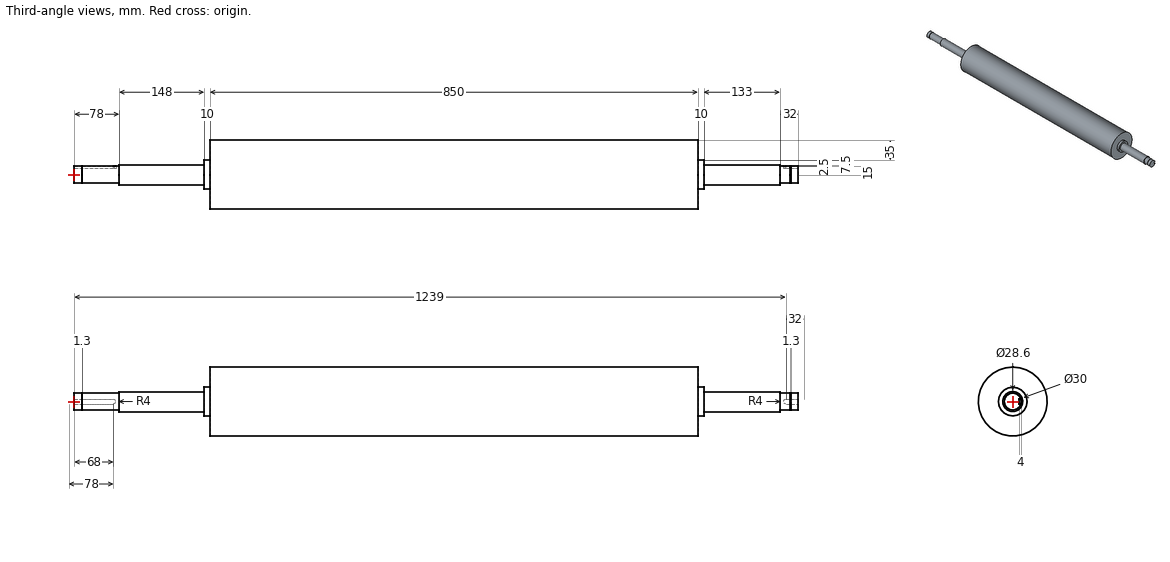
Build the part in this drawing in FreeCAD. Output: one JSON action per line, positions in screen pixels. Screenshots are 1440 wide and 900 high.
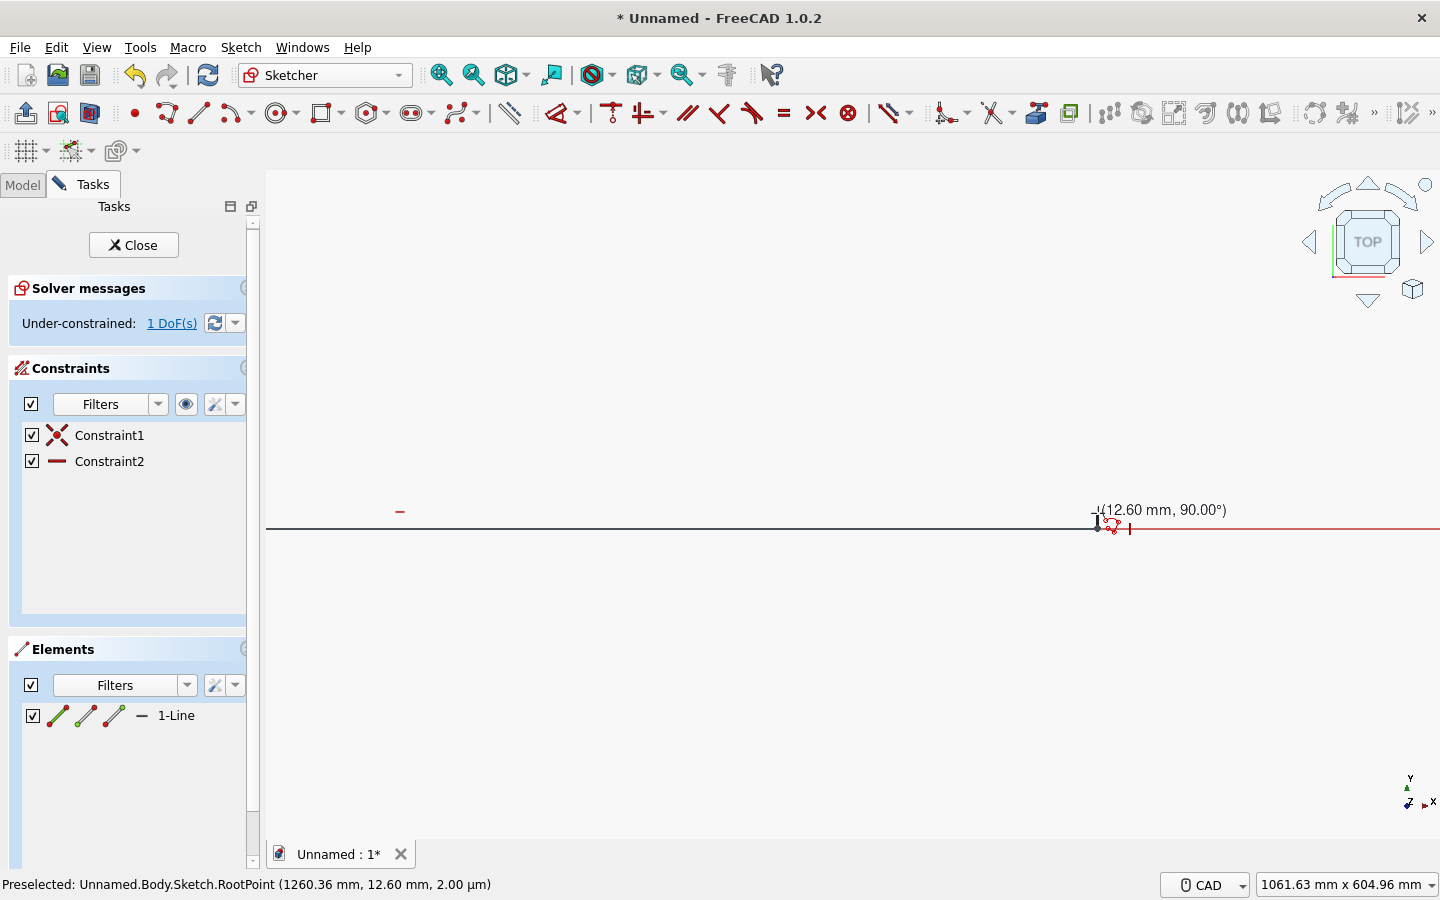
{"action": "left_click", "coordinate": [1097, 512]}
{"action": "left_click", "coordinate": [1062, 512]}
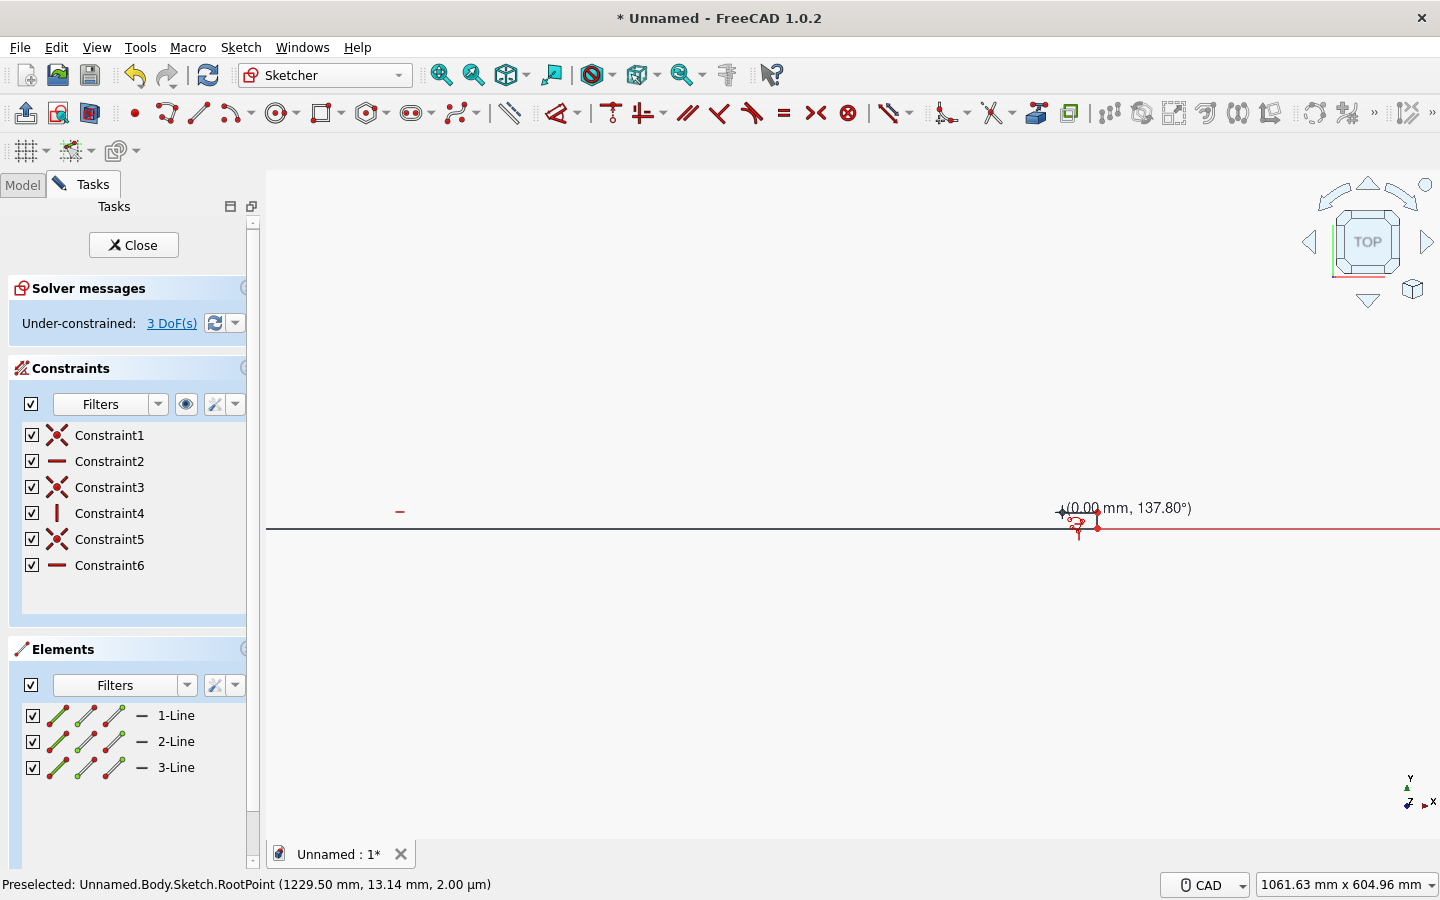
{"action": "scroll", "coordinate": [1062, 509], "scroll_direction": "up", "scroll_amount": 9}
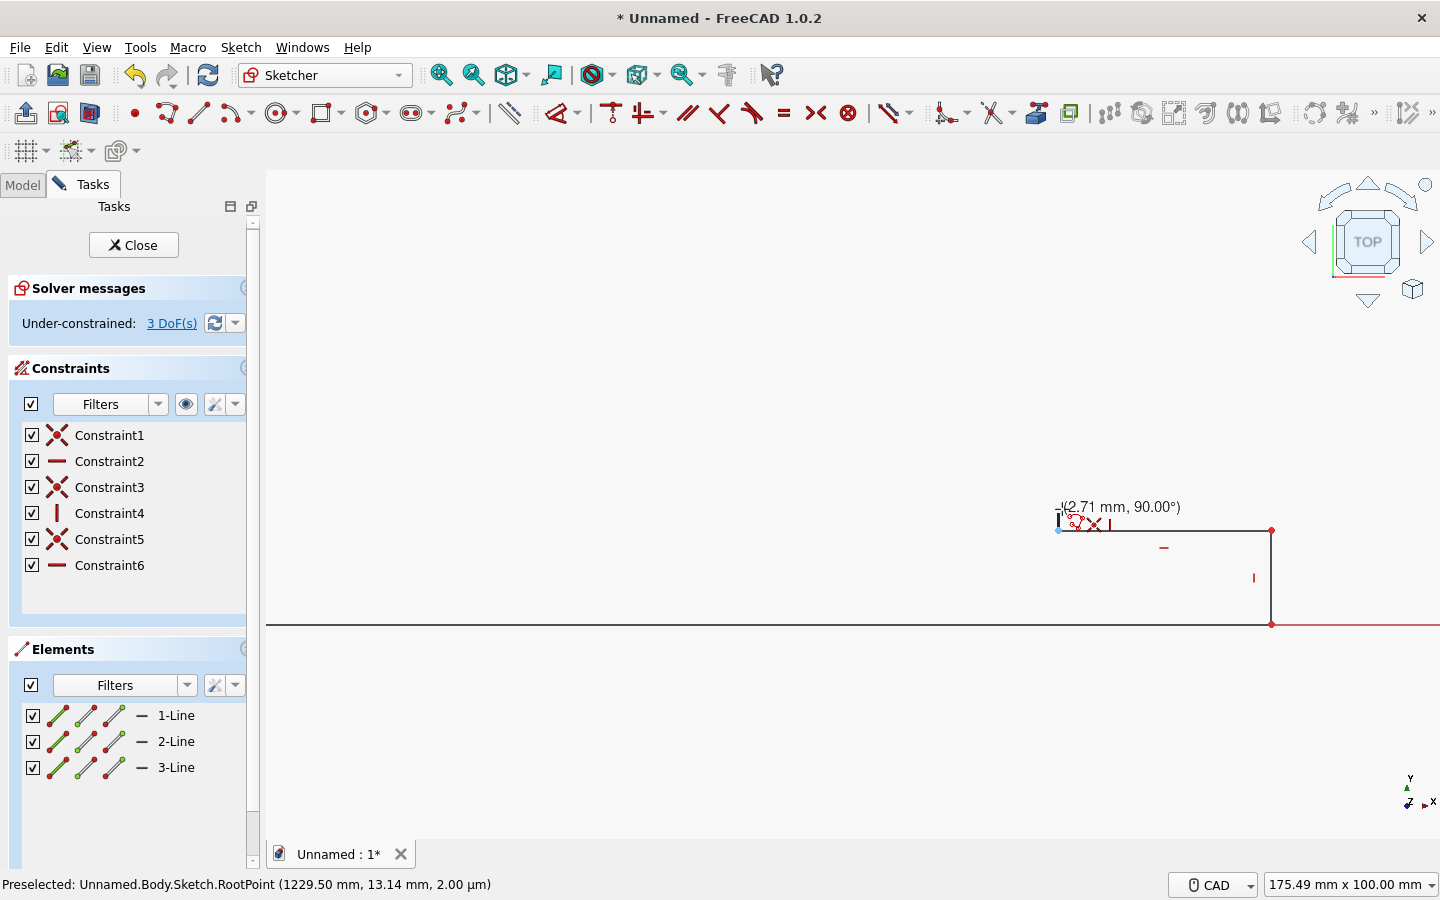
{"action": "left_click", "coordinate": [1059, 508]}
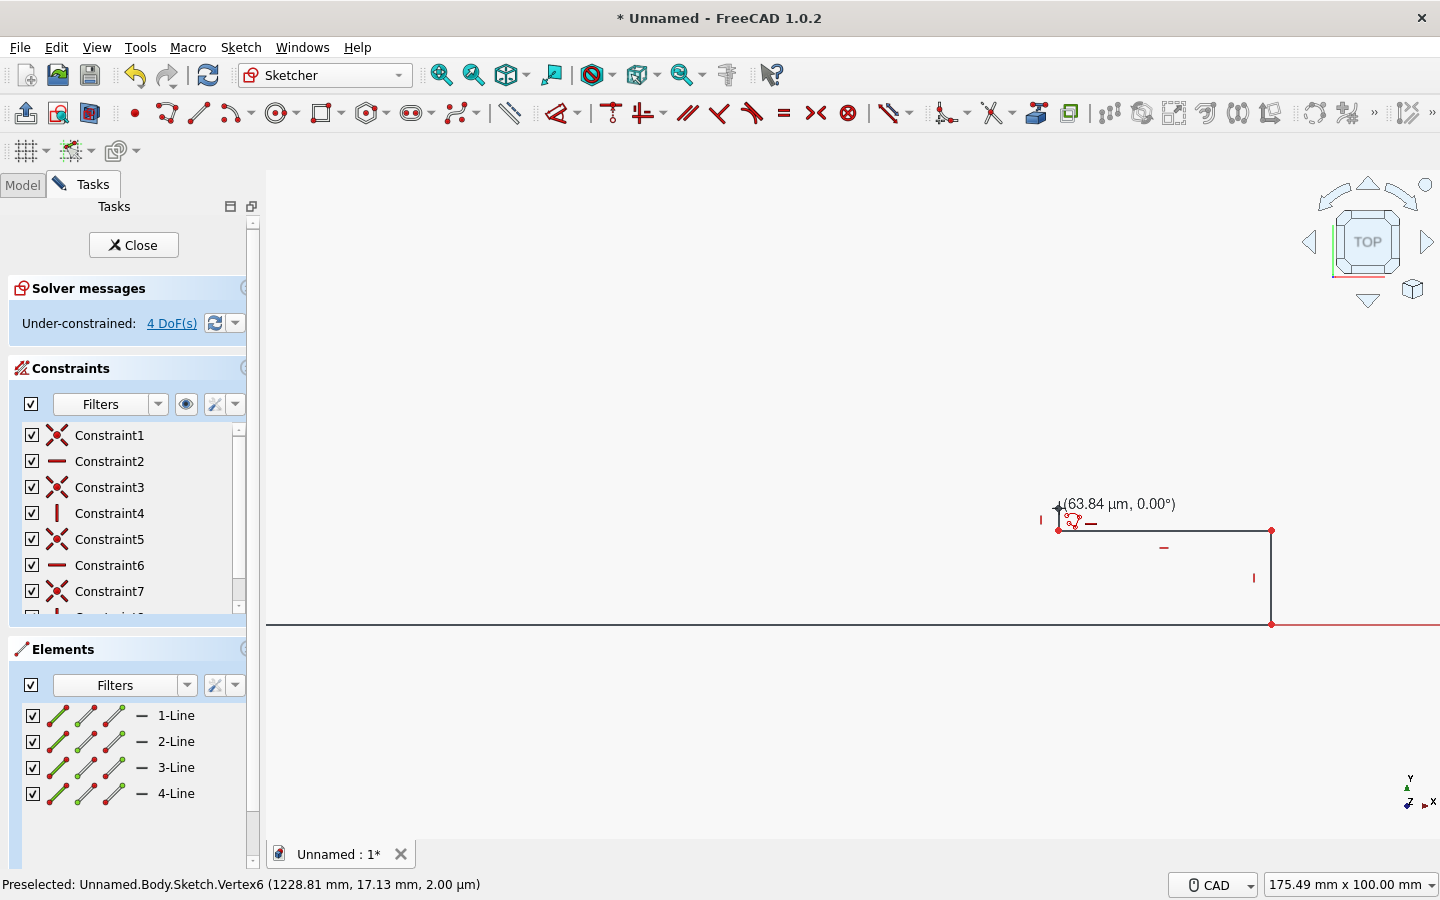
{"action": "scroll", "coordinate": [1084, 511], "scroll_direction": "down", "scroll_amount": 13}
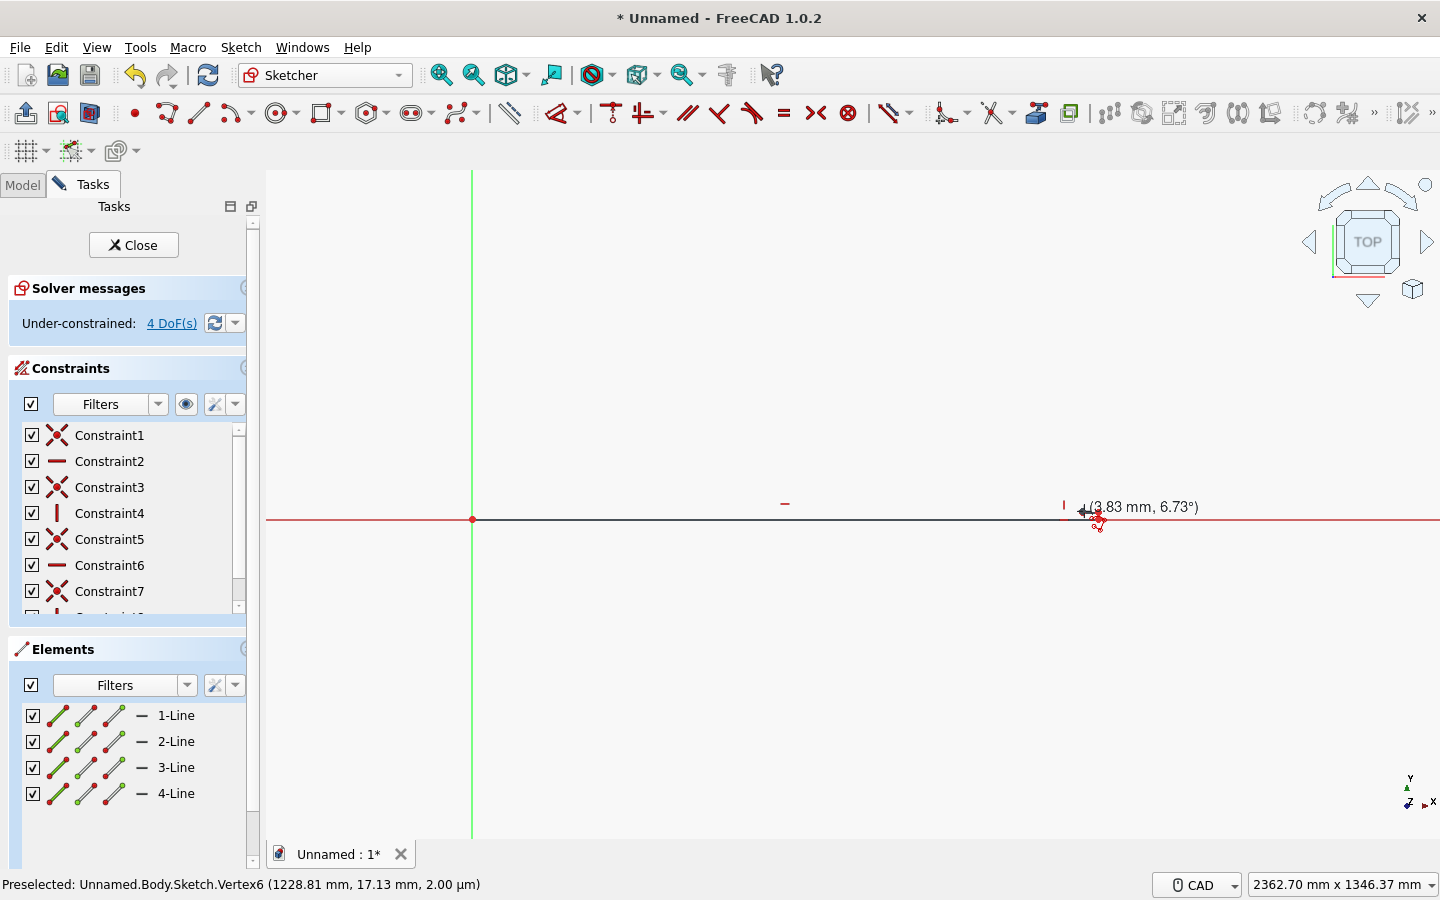
{"action": "scroll", "coordinate": [1017, 511], "scroll_direction": "up", "scroll_amount": 4}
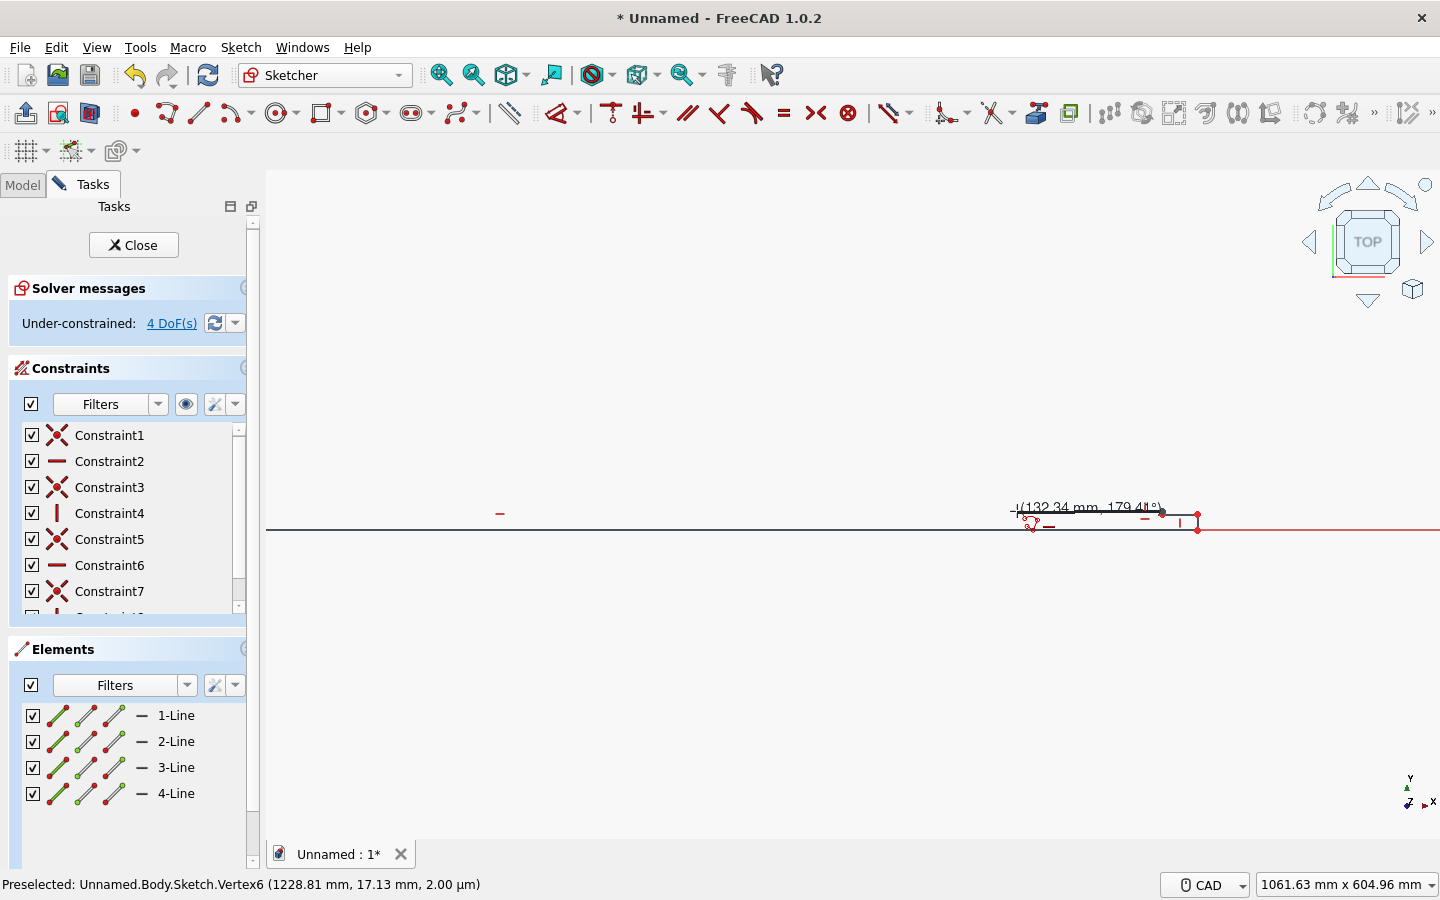
{"action": "left_click", "coordinate": [1016, 511]}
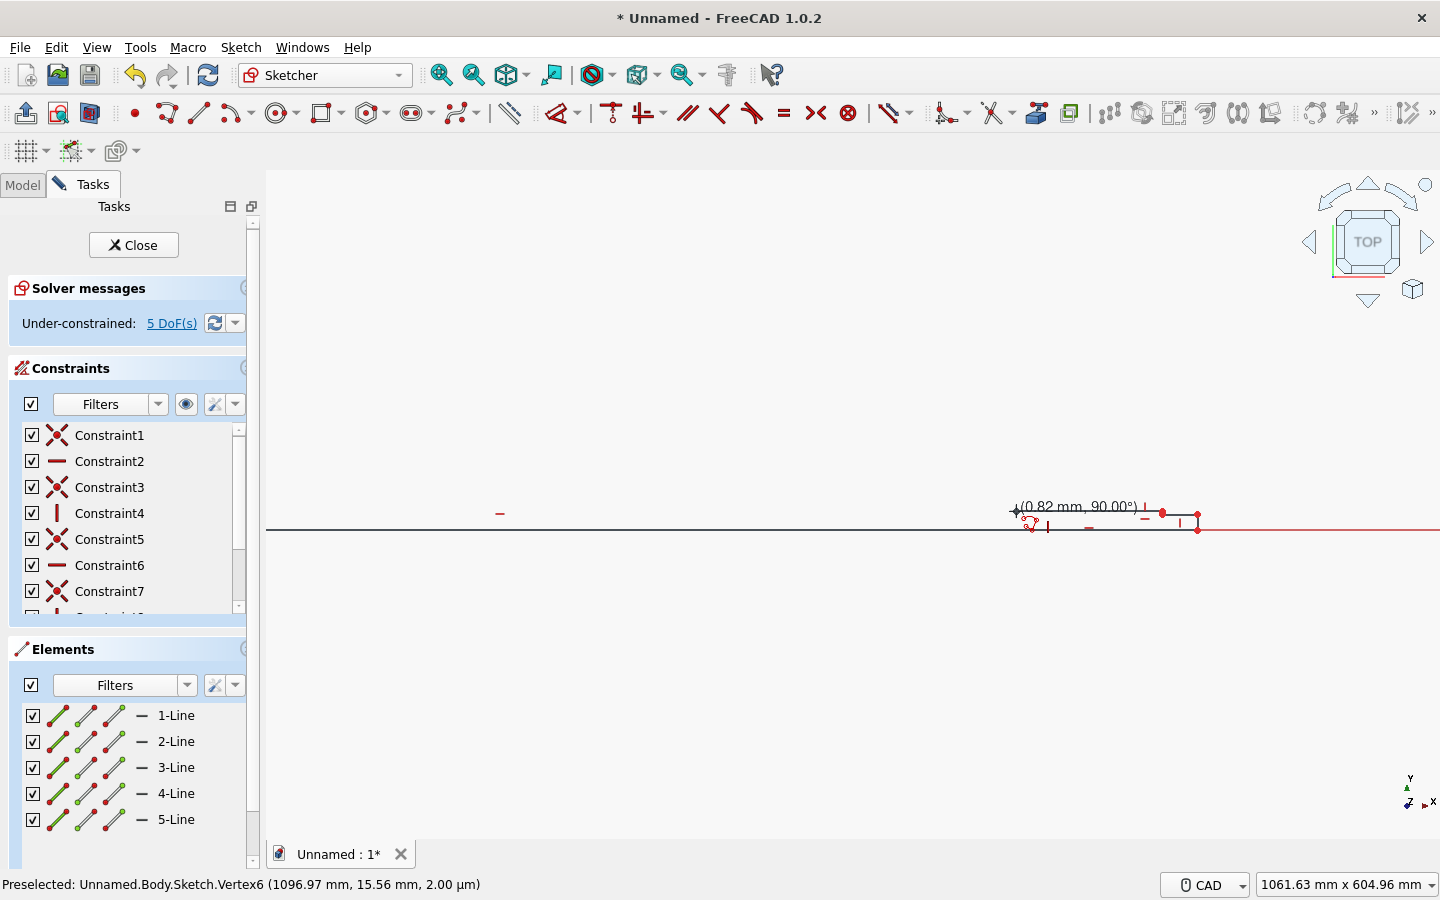
{"action": "scroll", "coordinate": [1016, 503], "scroll_direction": "up", "scroll_amount": 4}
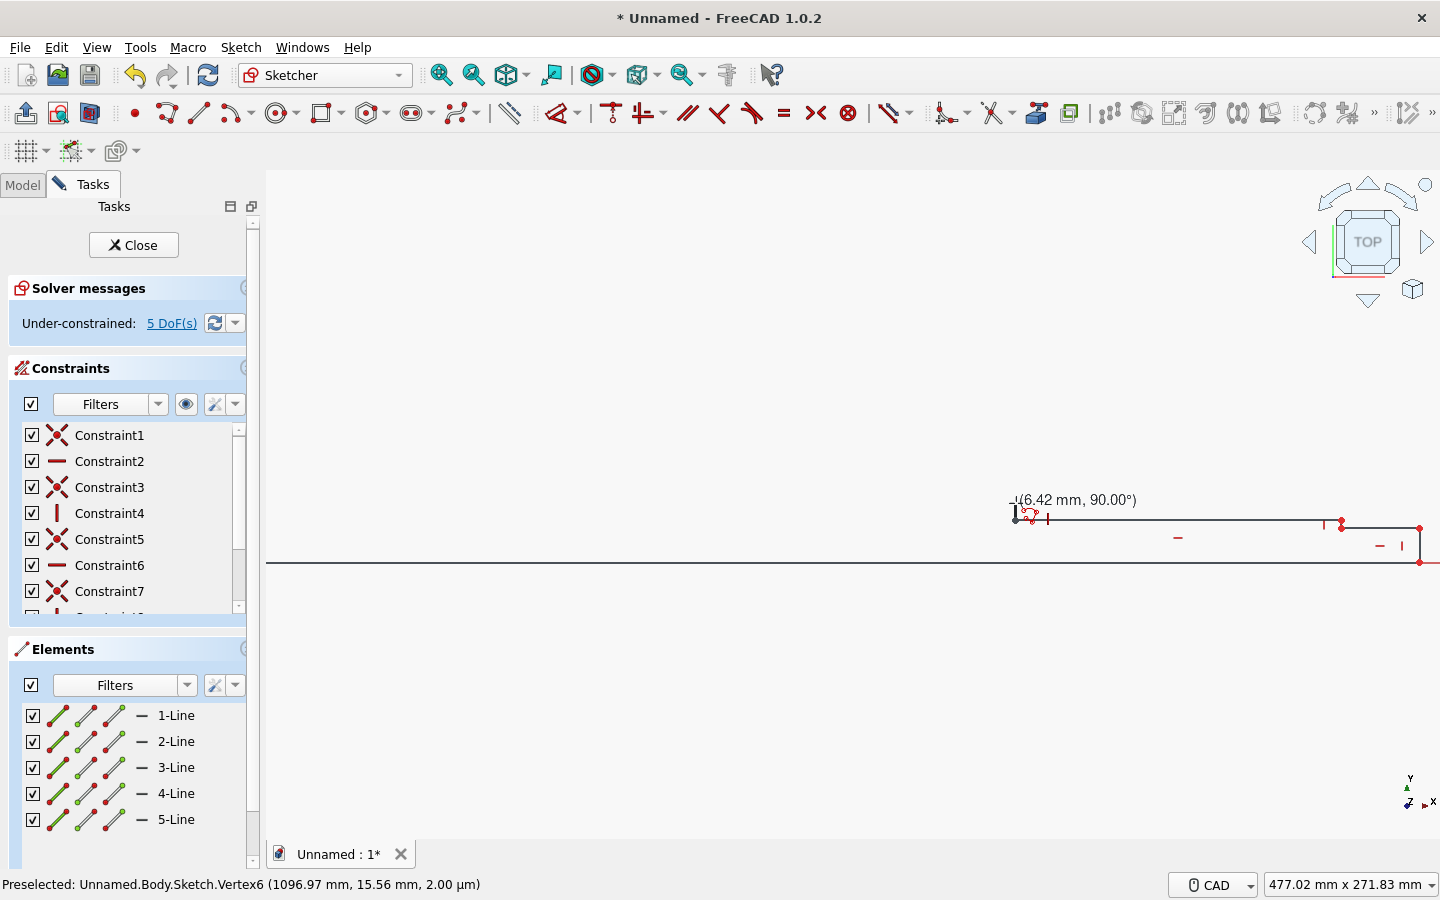
{"action": "left_click", "coordinate": [1015, 501]}
{"action": "left_click", "coordinate": [990, 501]}